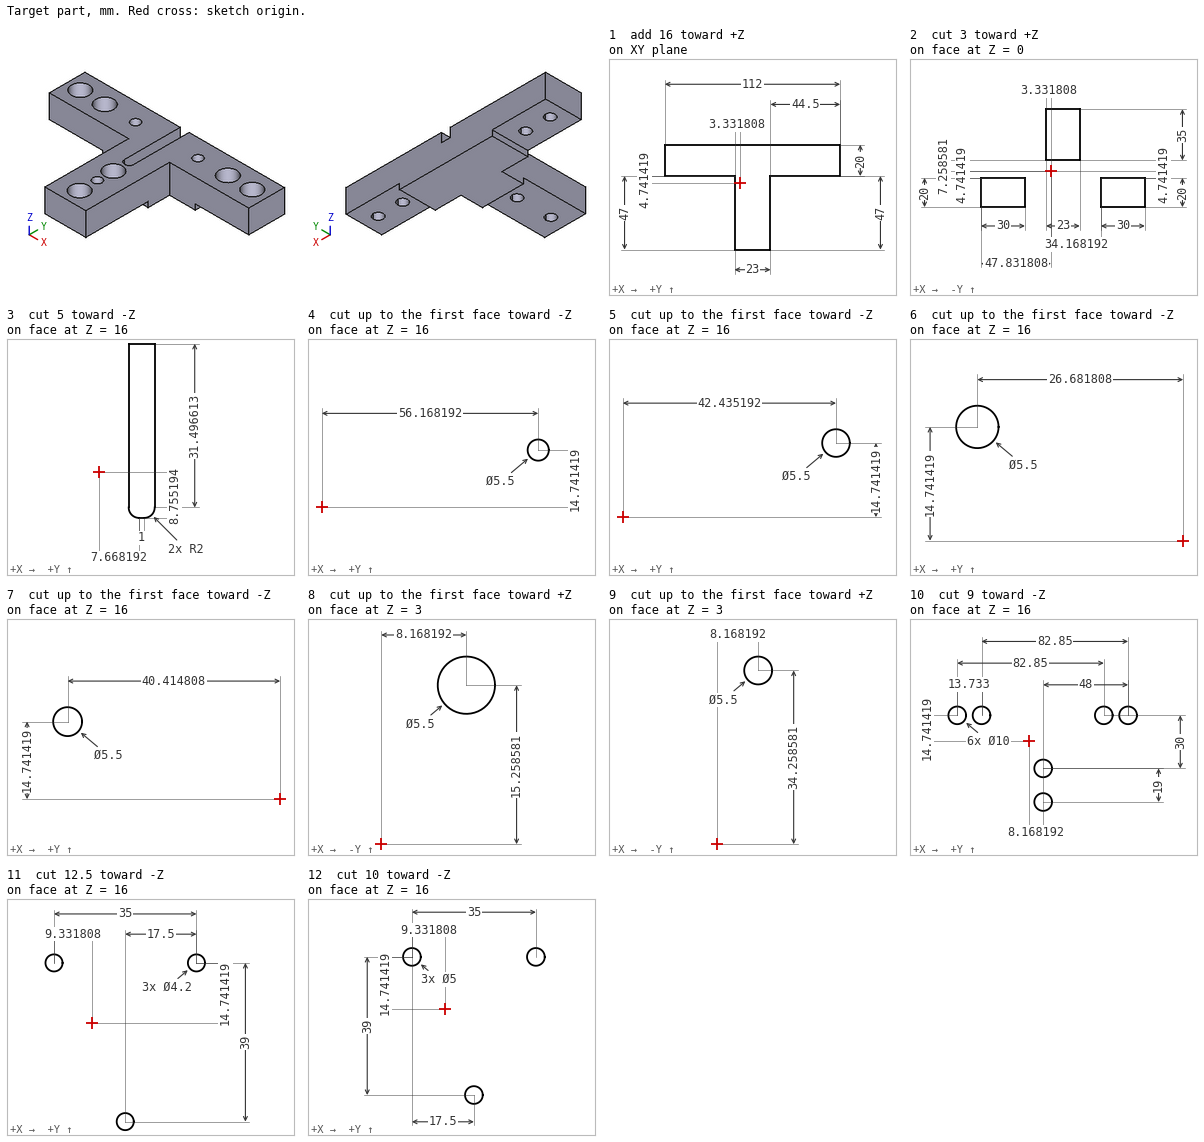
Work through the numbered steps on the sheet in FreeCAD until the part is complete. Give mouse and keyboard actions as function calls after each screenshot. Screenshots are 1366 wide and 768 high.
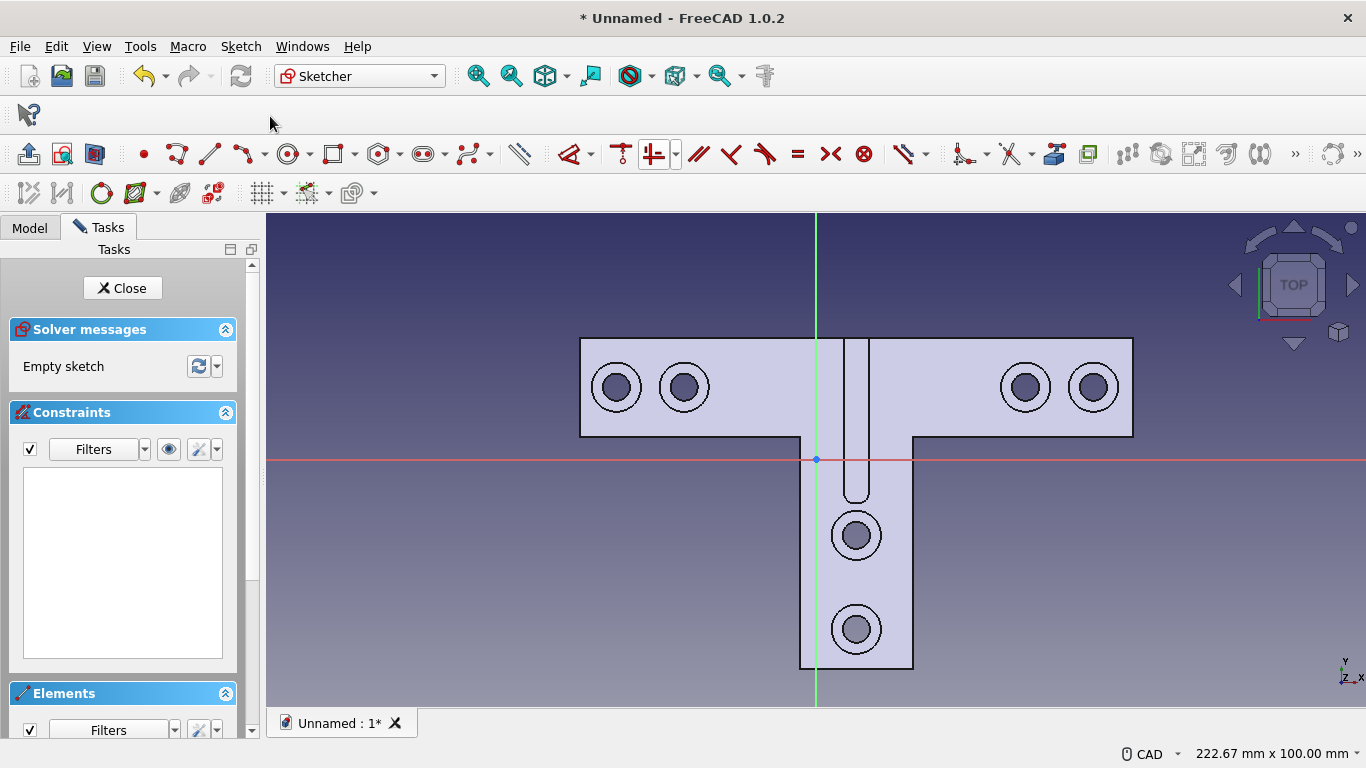
scroll(1078, 531, up, 2)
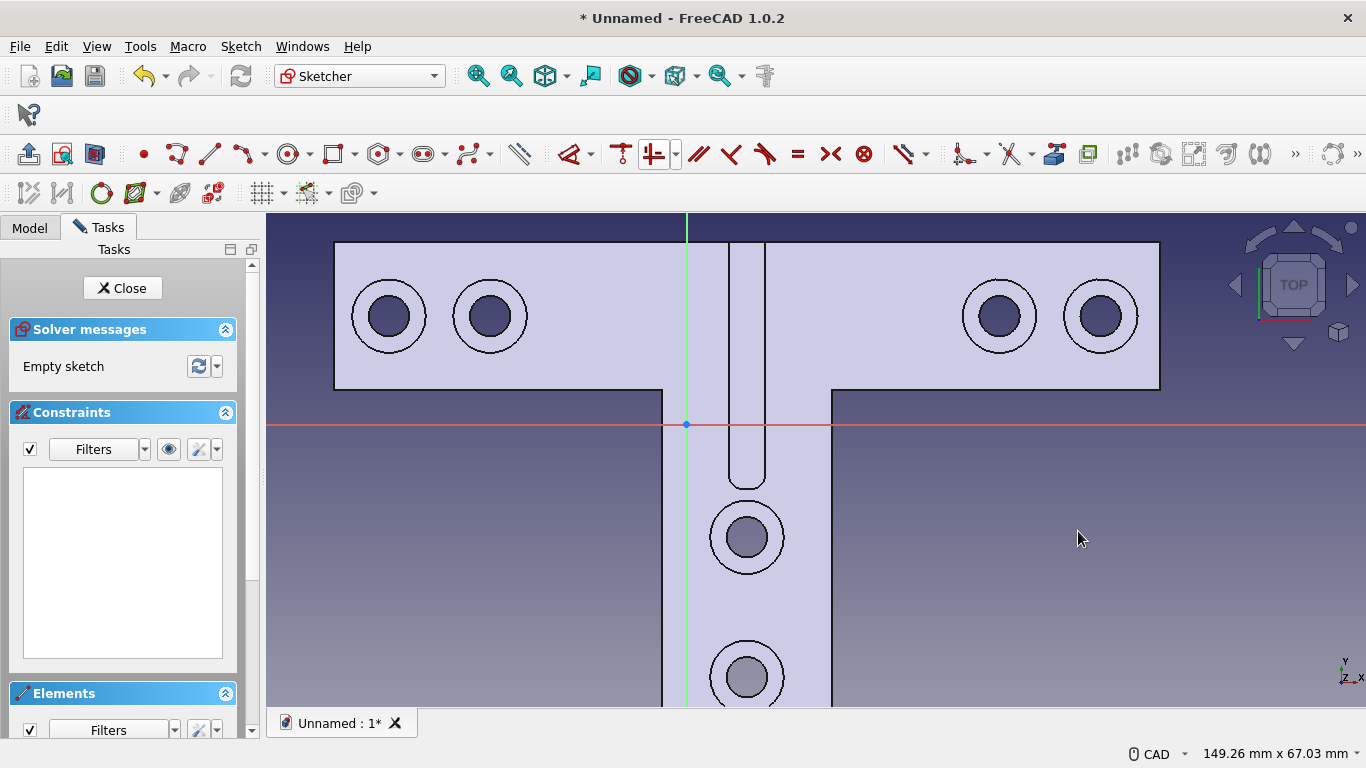
click(288, 154)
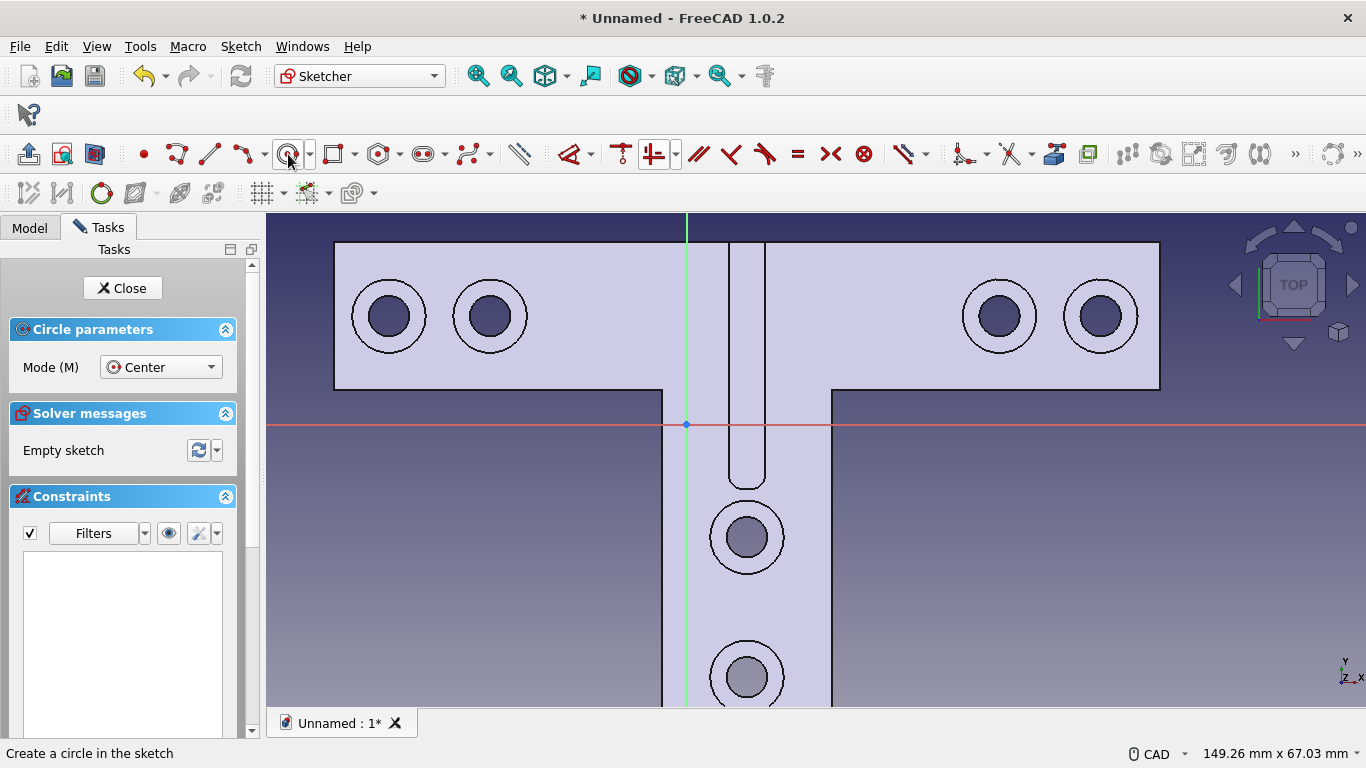
scroll(876, 316, up, 2)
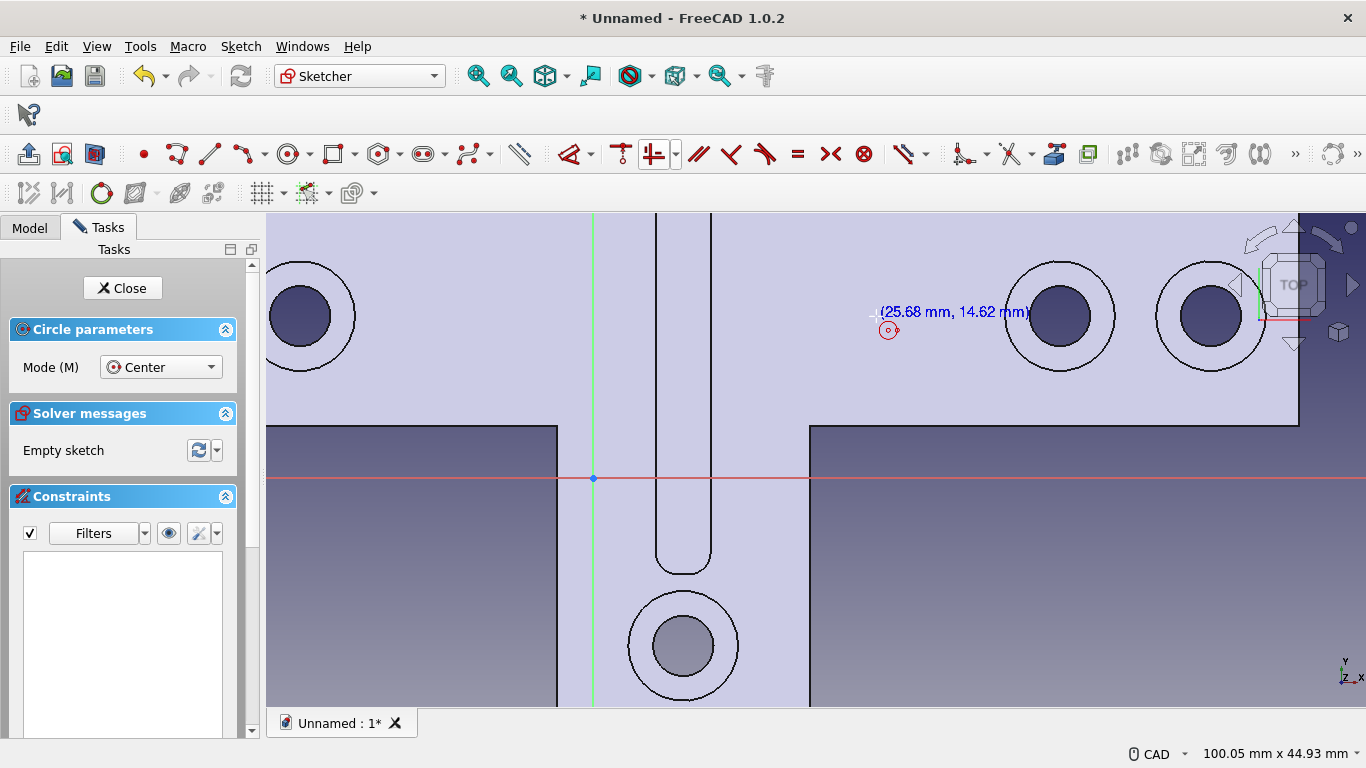
click(876, 316)
move(892, 300)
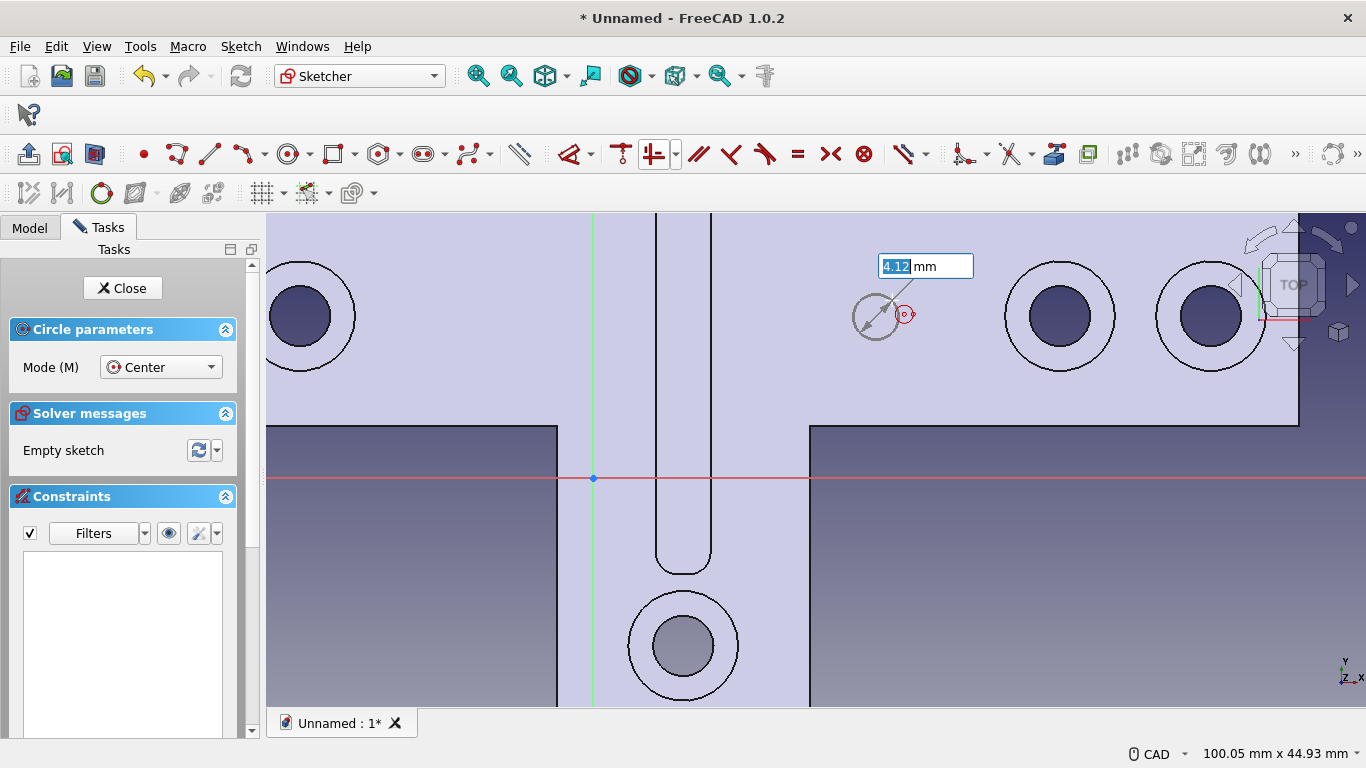
text(4.2)
key(Return)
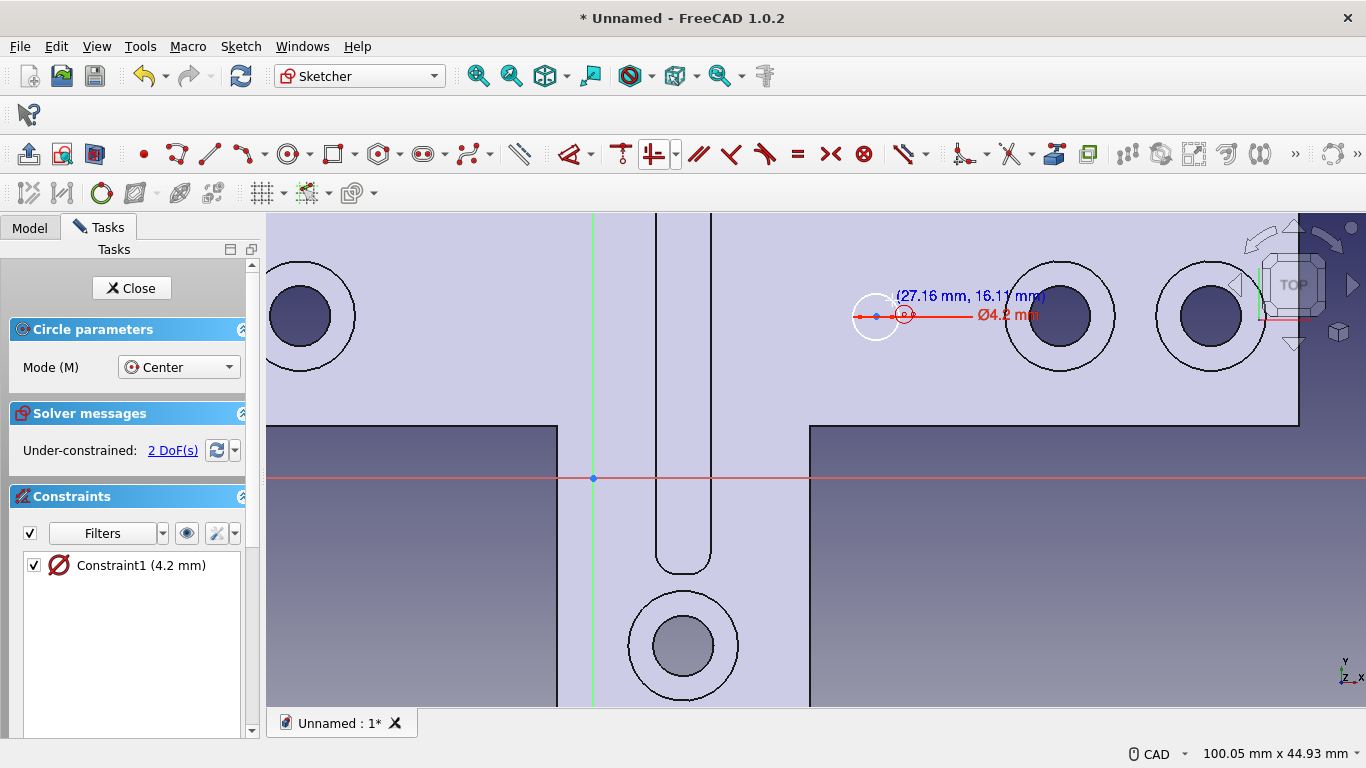
click(491, 316)
move(507, 300)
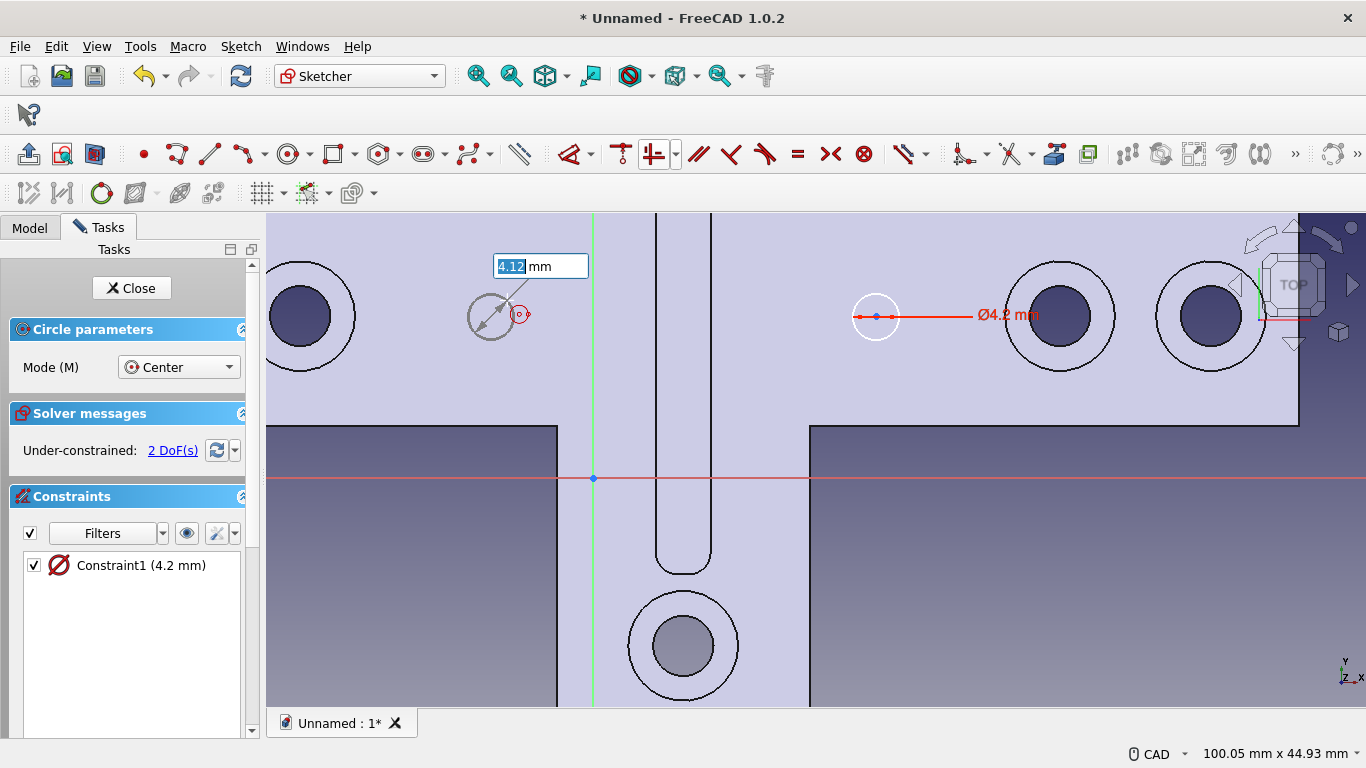
text(4.2)
key(Return)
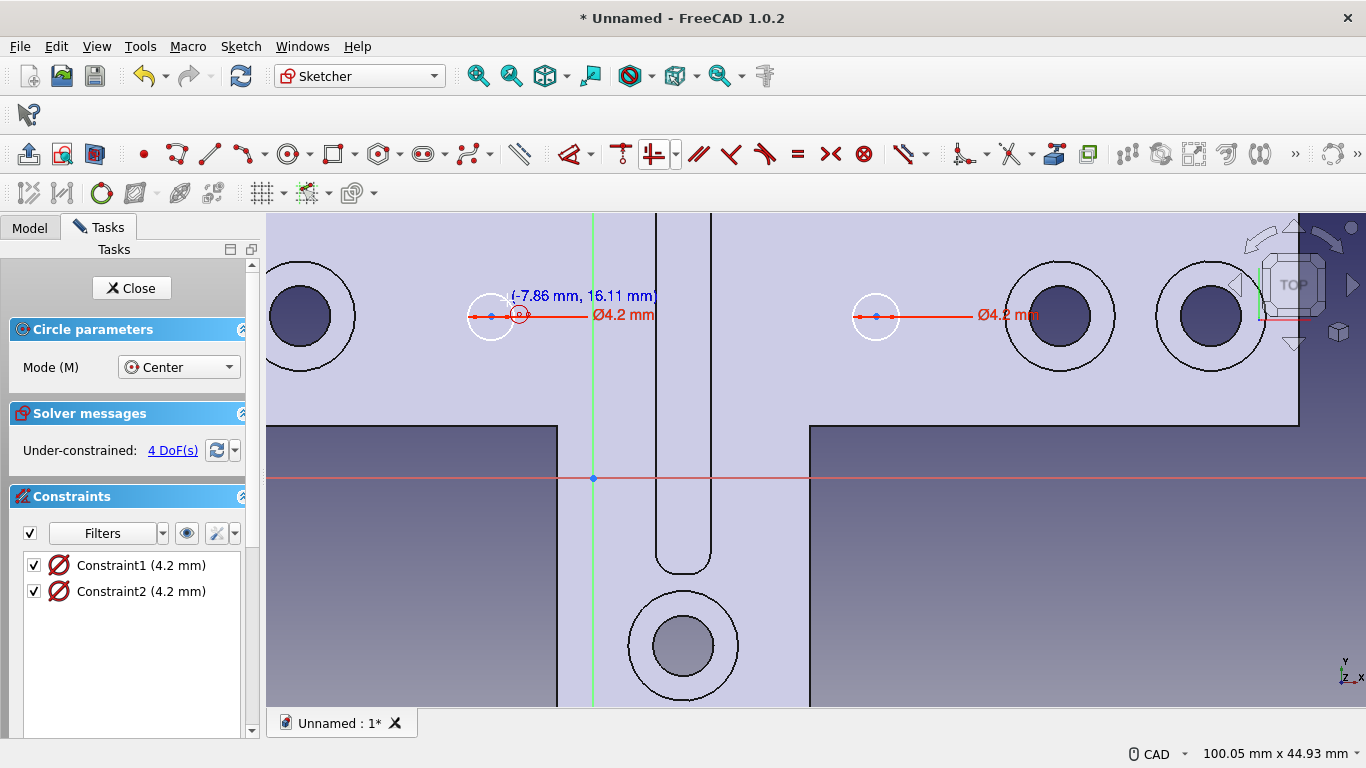
scroll(878, 317, down, 2)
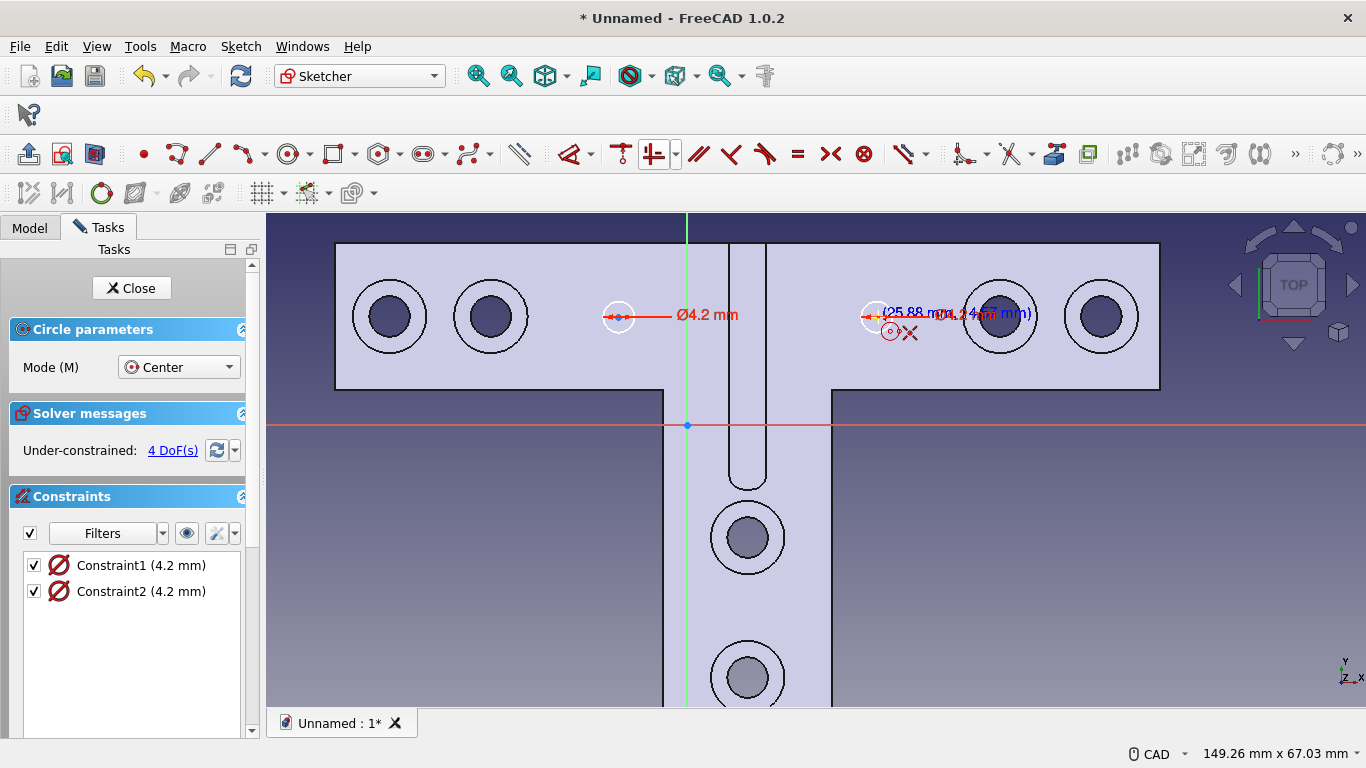
scroll(748, 604, up, 2)